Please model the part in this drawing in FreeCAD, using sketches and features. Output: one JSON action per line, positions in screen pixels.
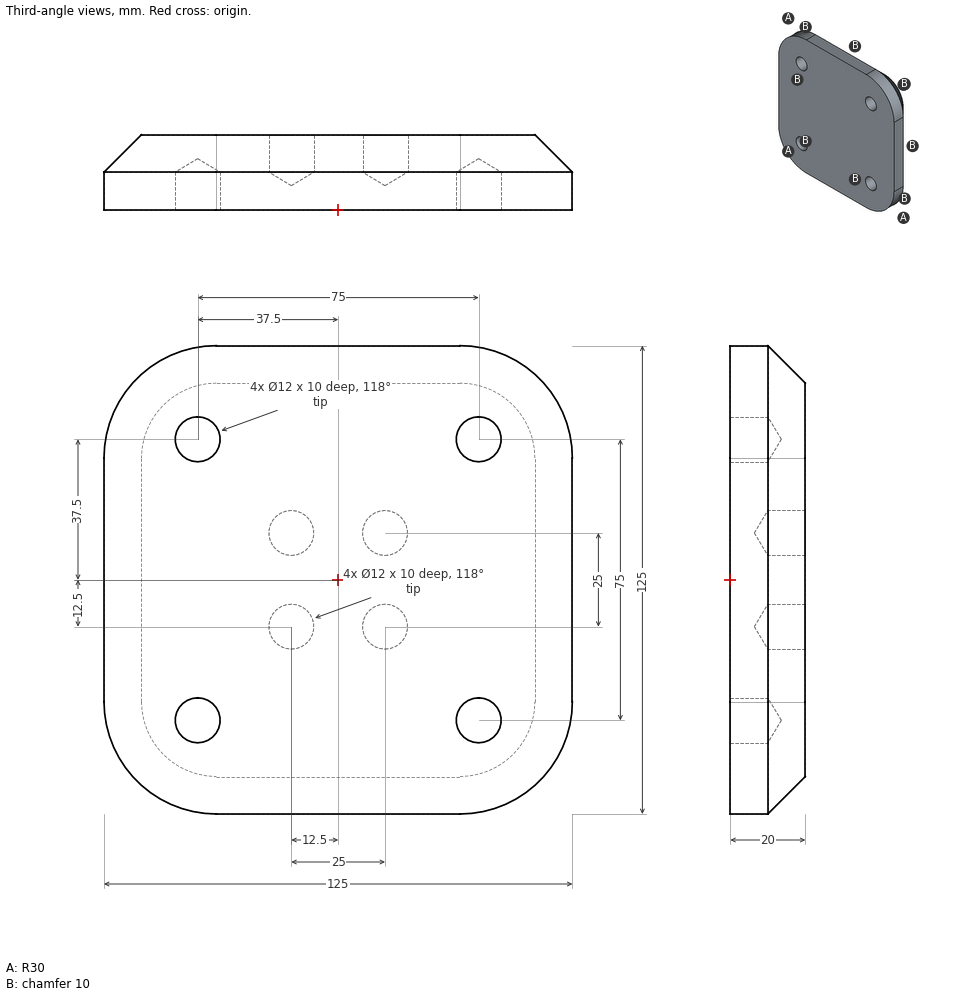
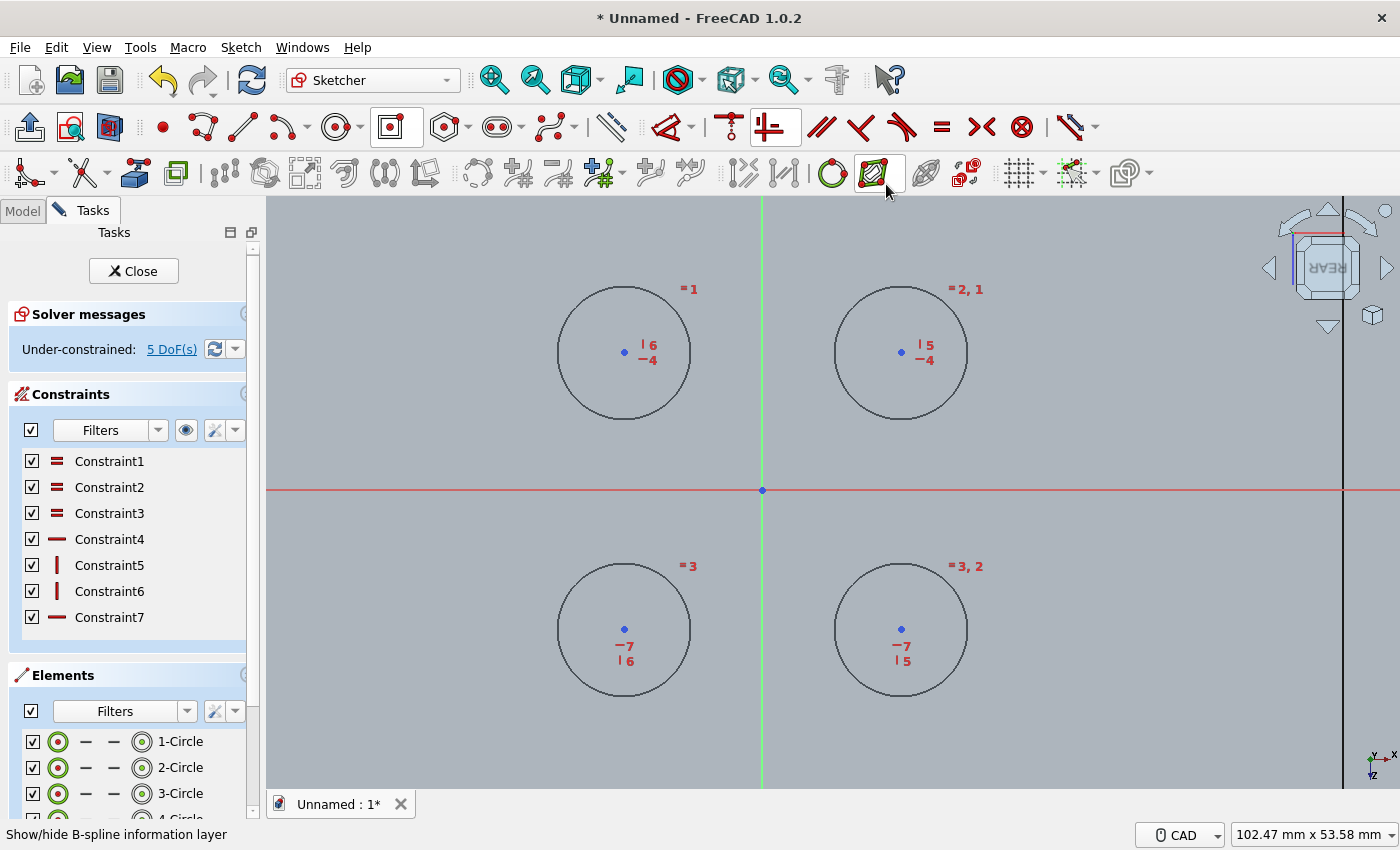
{"action": "key", "text": "d"}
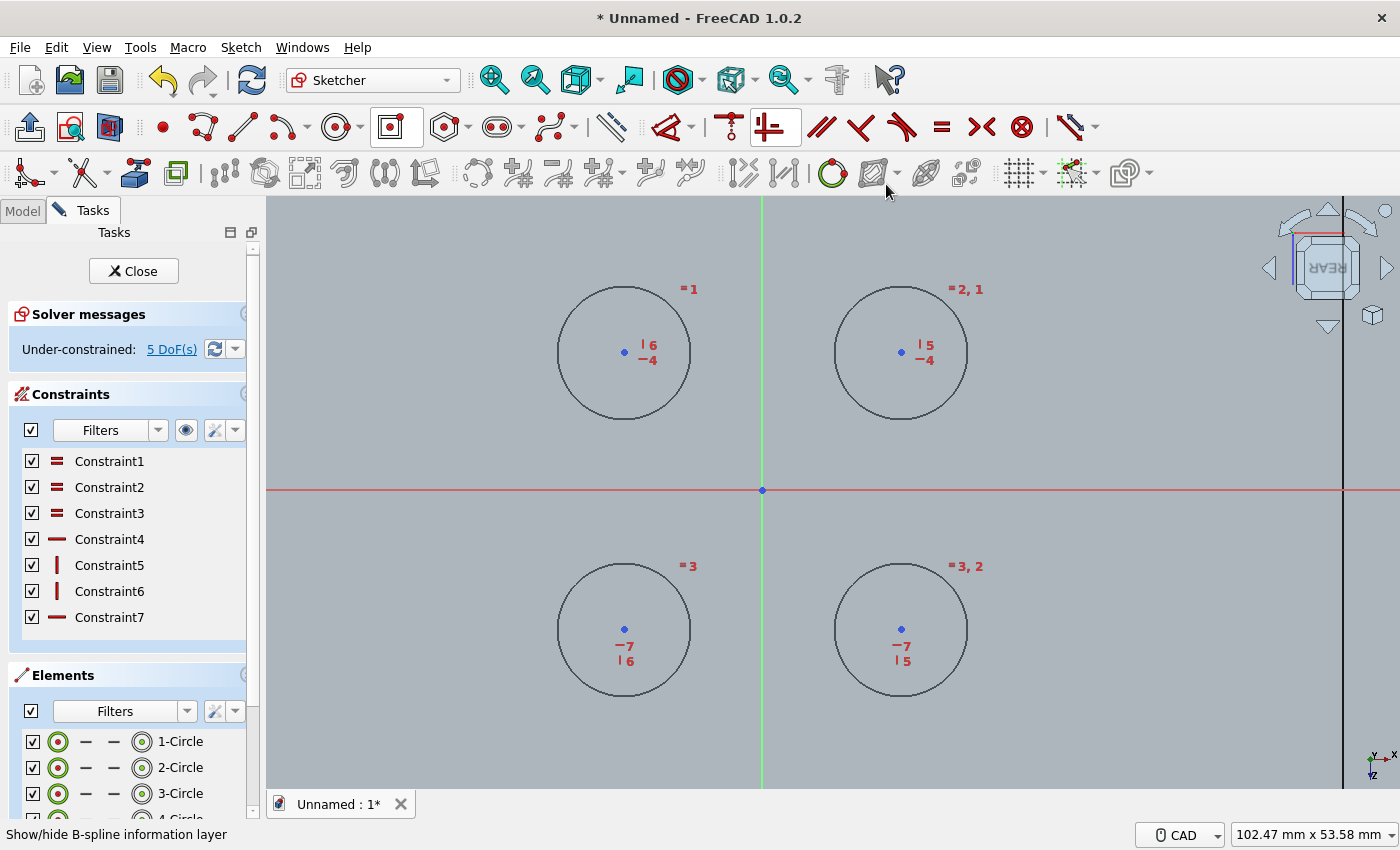
{"action": "left_click", "coordinate": [671, 306]}
{"action": "left_click", "coordinate": [694, 283]}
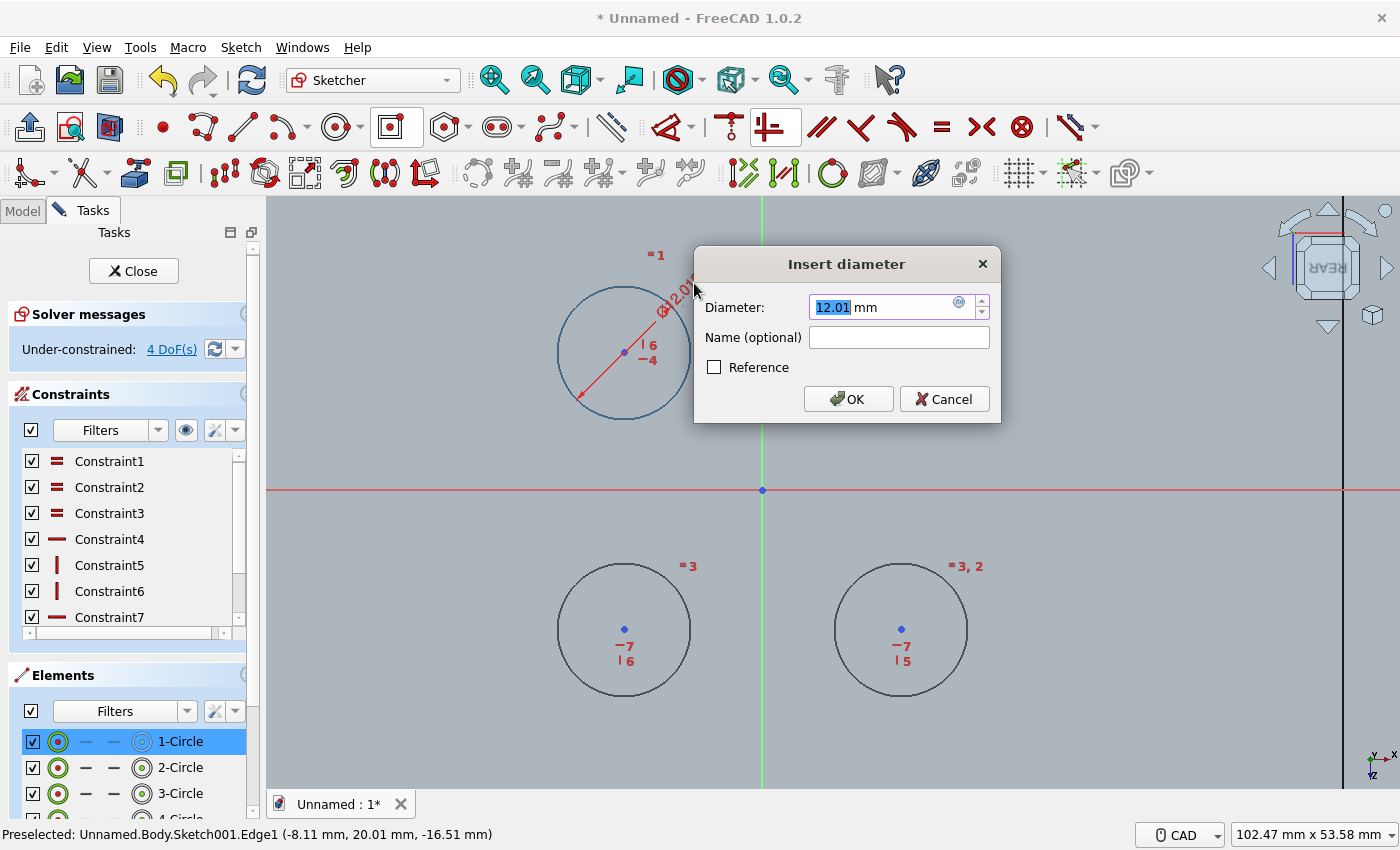
{"action": "type", "text": "12"}
{"action": "key", "text": "Return"}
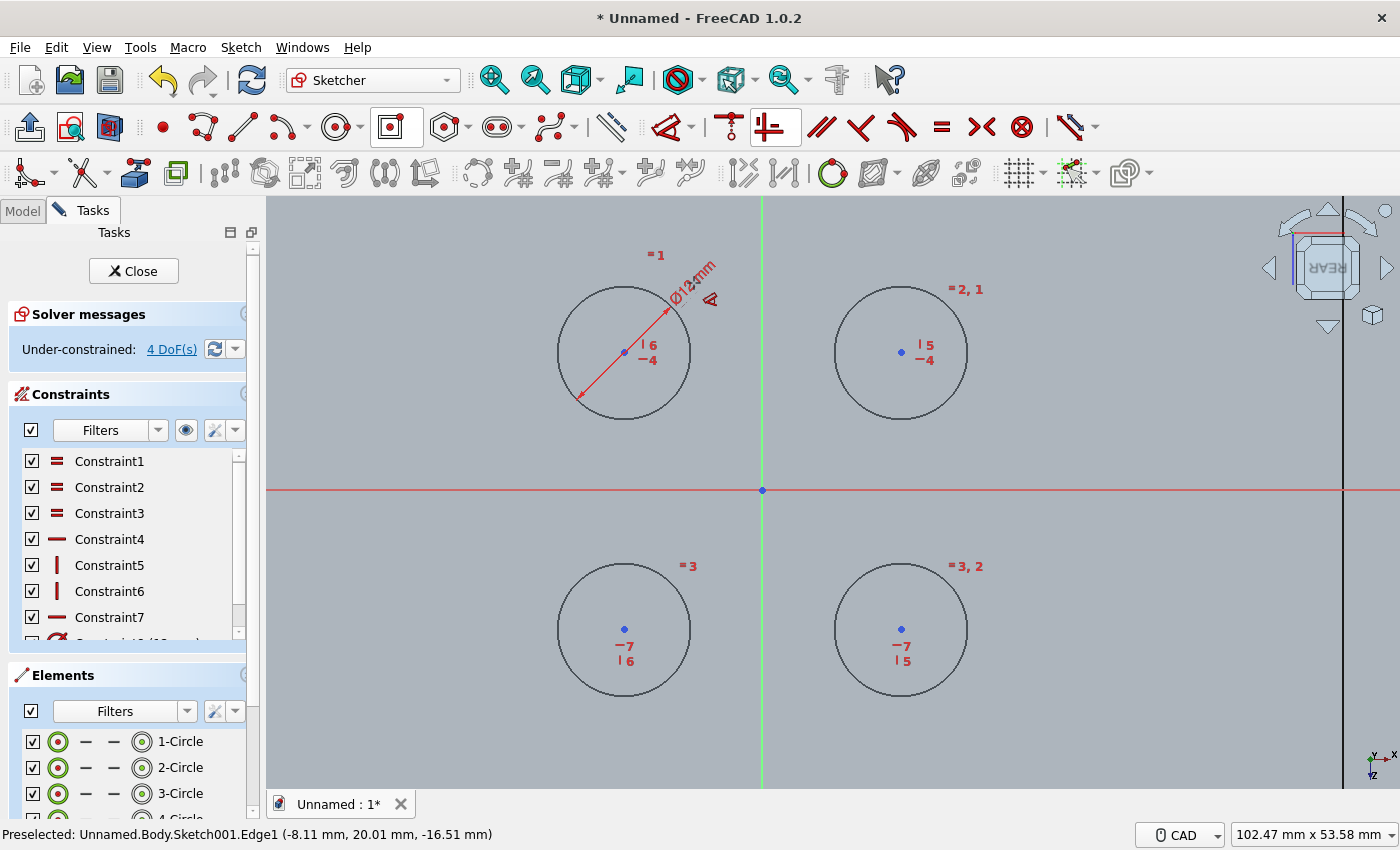
{"action": "left_click", "coordinate": [624, 353]}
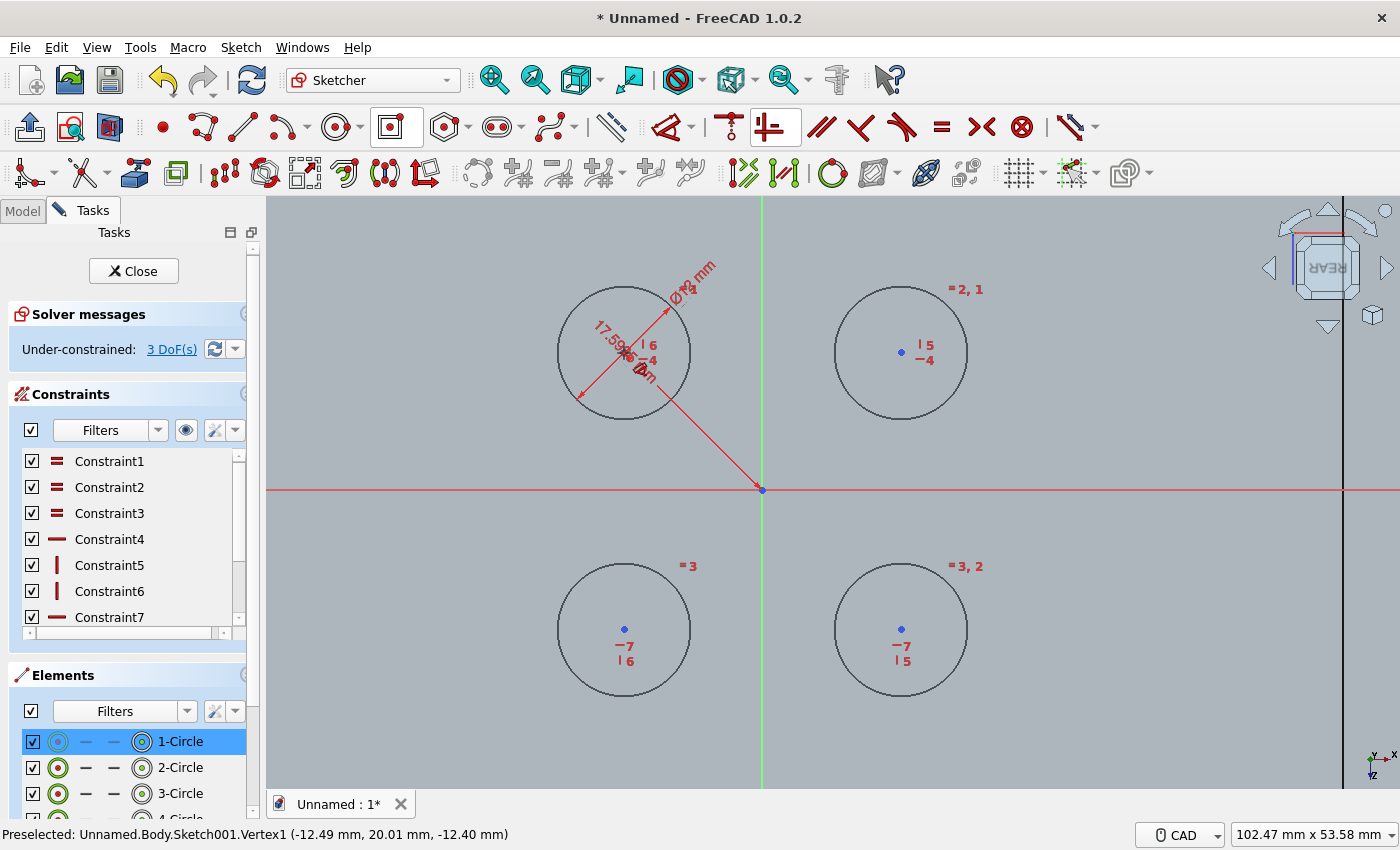
{"action": "left_click", "coordinate": [901, 353]}
{"action": "left_click", "coordinate": [699, 319]}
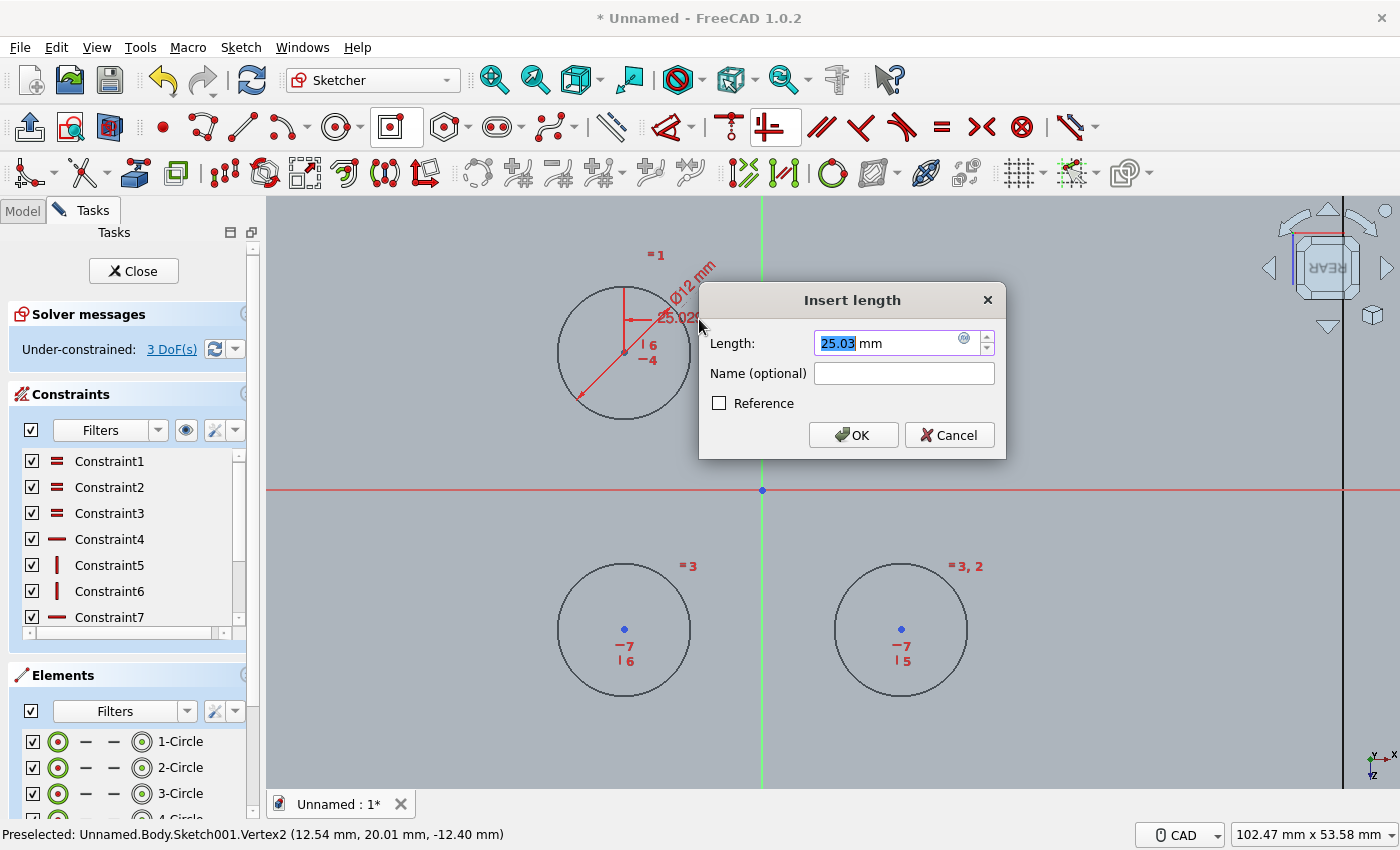
{"action": "type", "text": "25"}
{"action": "key", "text": "Return"}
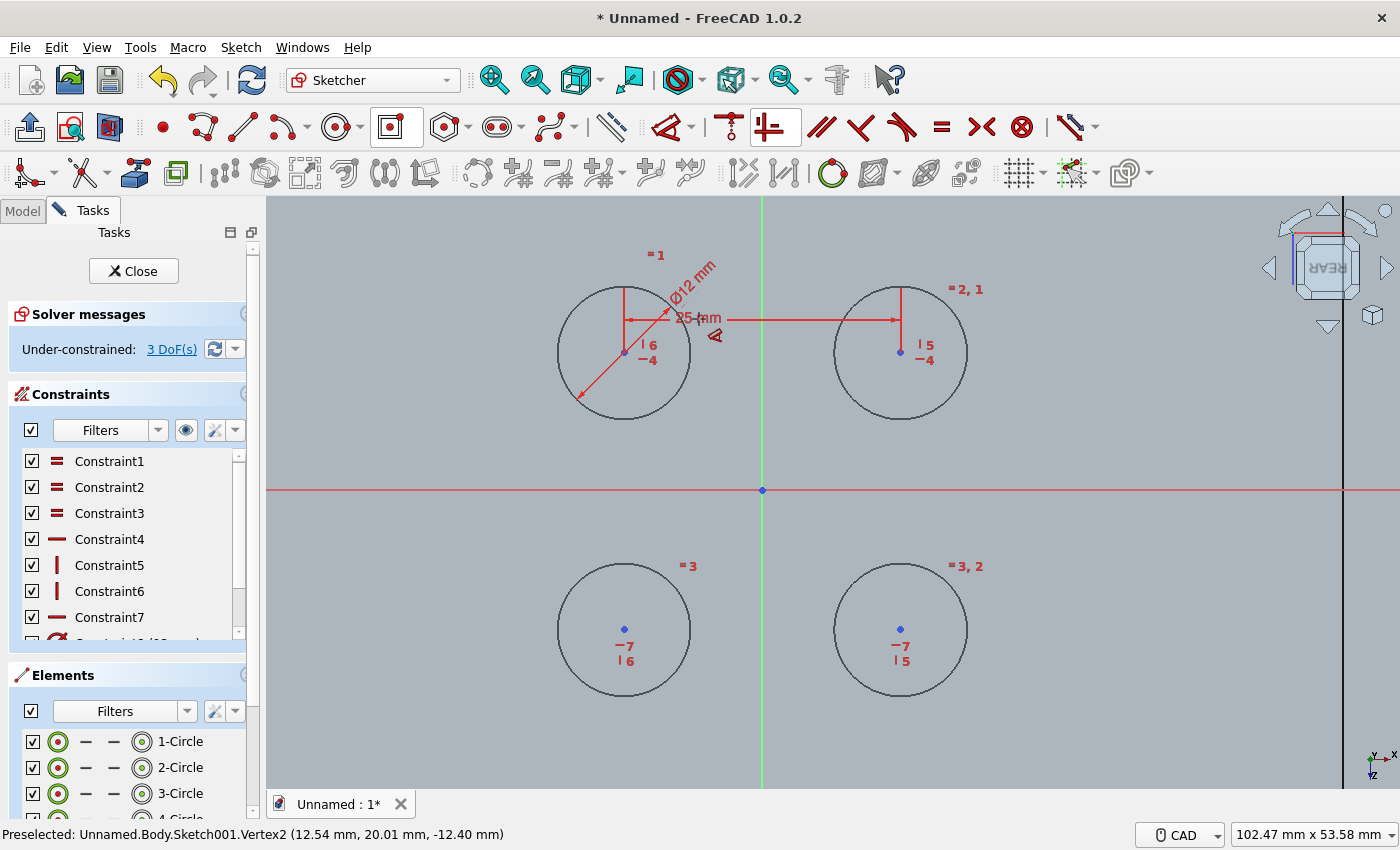
{"action": "left_click", "coordinate": [901, 353]}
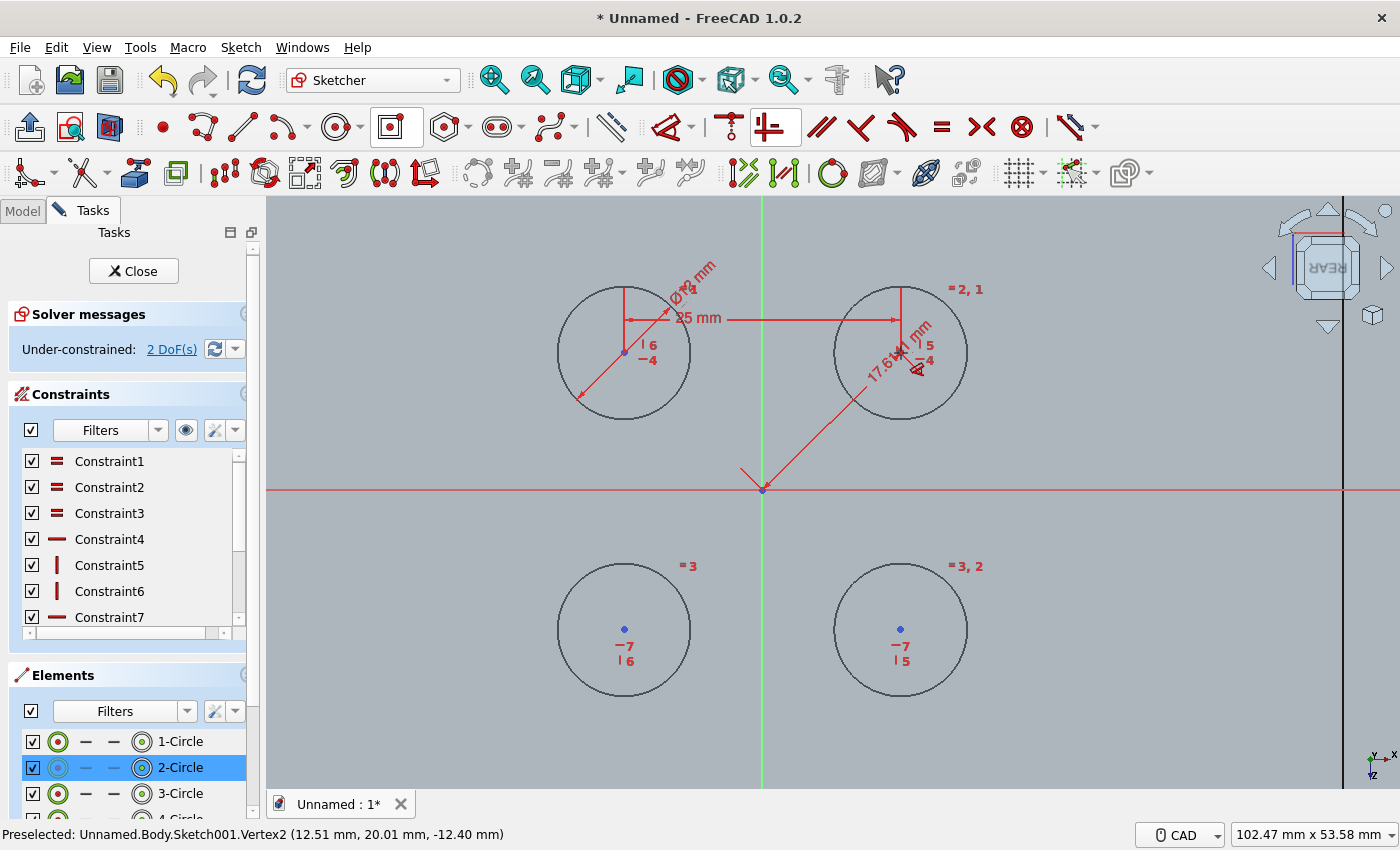
{"action": "left_click", "coordinate": [901, 630]}
{"action": "left_click", "coordinate": [935, 428]}